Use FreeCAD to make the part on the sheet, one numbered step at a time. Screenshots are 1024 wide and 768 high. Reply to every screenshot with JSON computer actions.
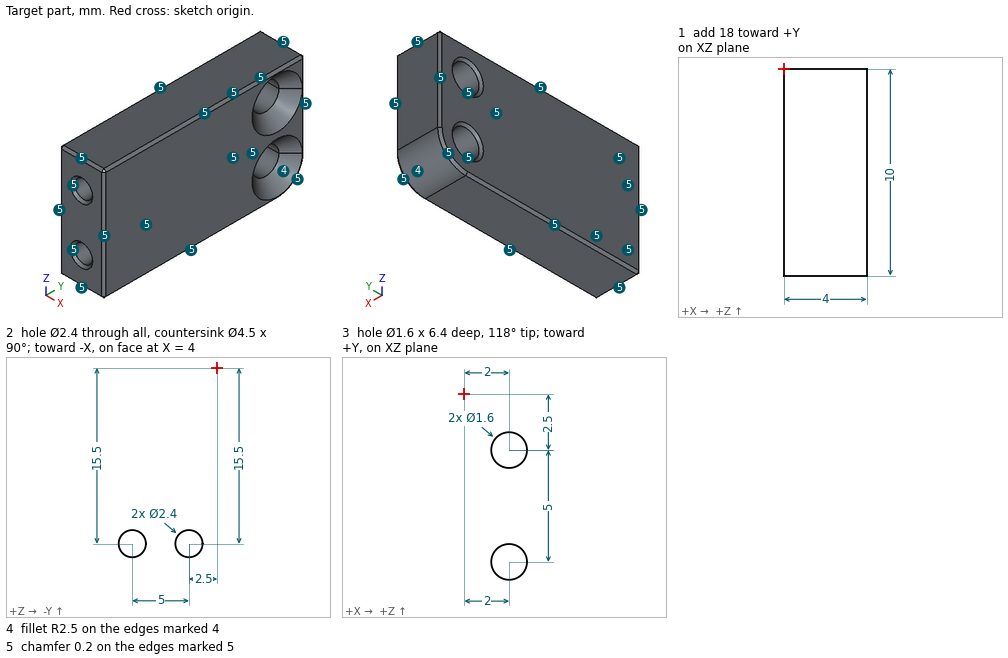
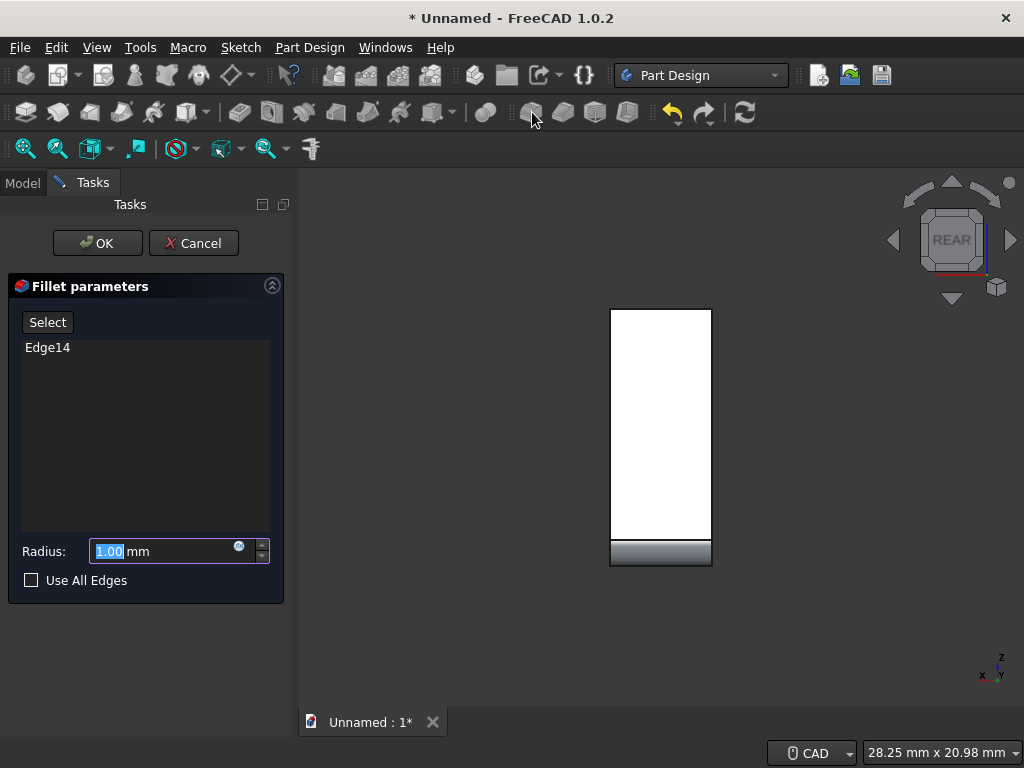
{"action": "type", "text": "2.5"}
{"action": "key", "text": "Tab"}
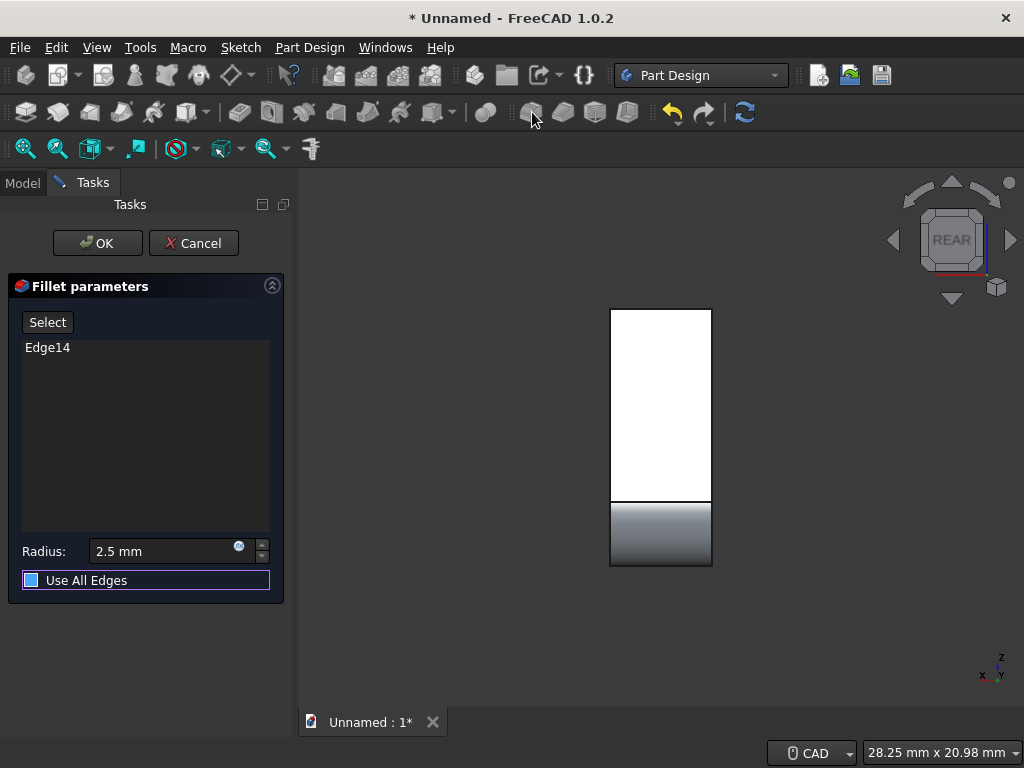
{"action": "left_click", "coordinate": [98, 243]}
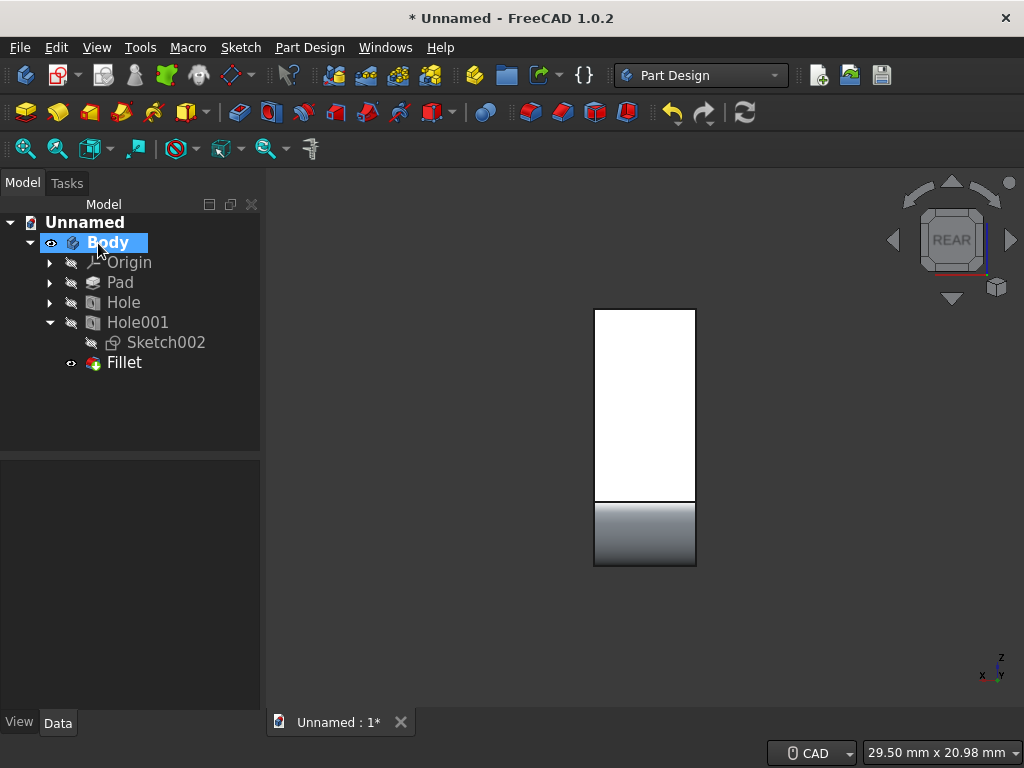
{"action": "left_click", "coordinate": [594, 404]}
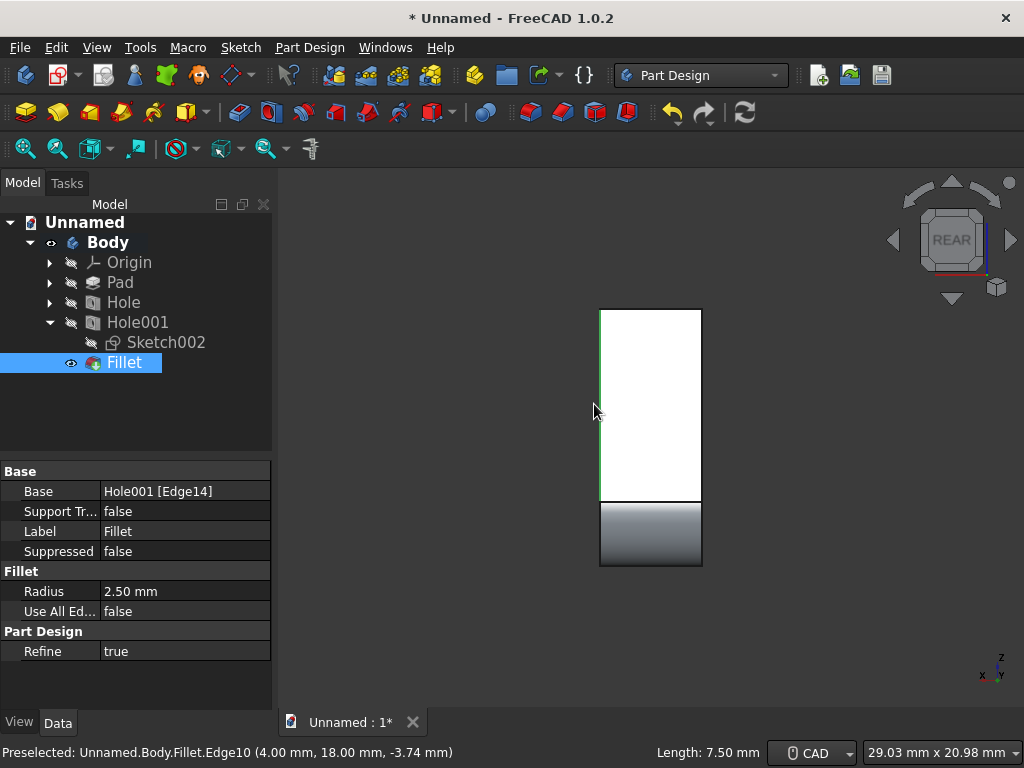
{"action": "left_click", "coordinate": [600, 546], "text": "ctrl"}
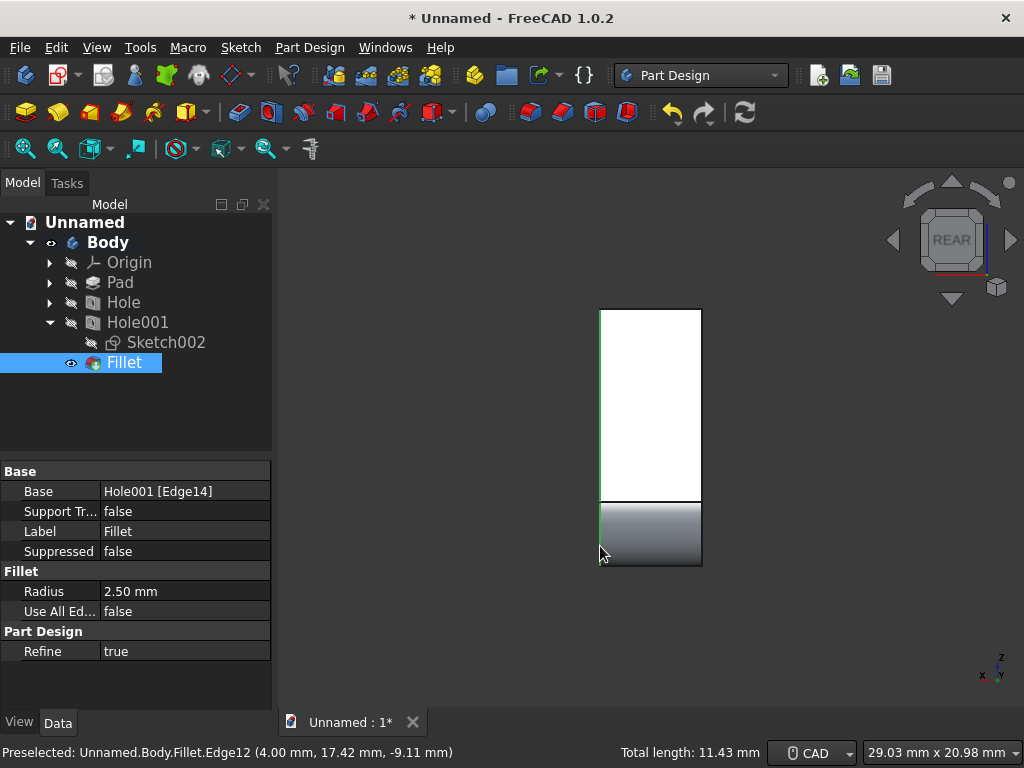
{"action": "key", "text": "0"}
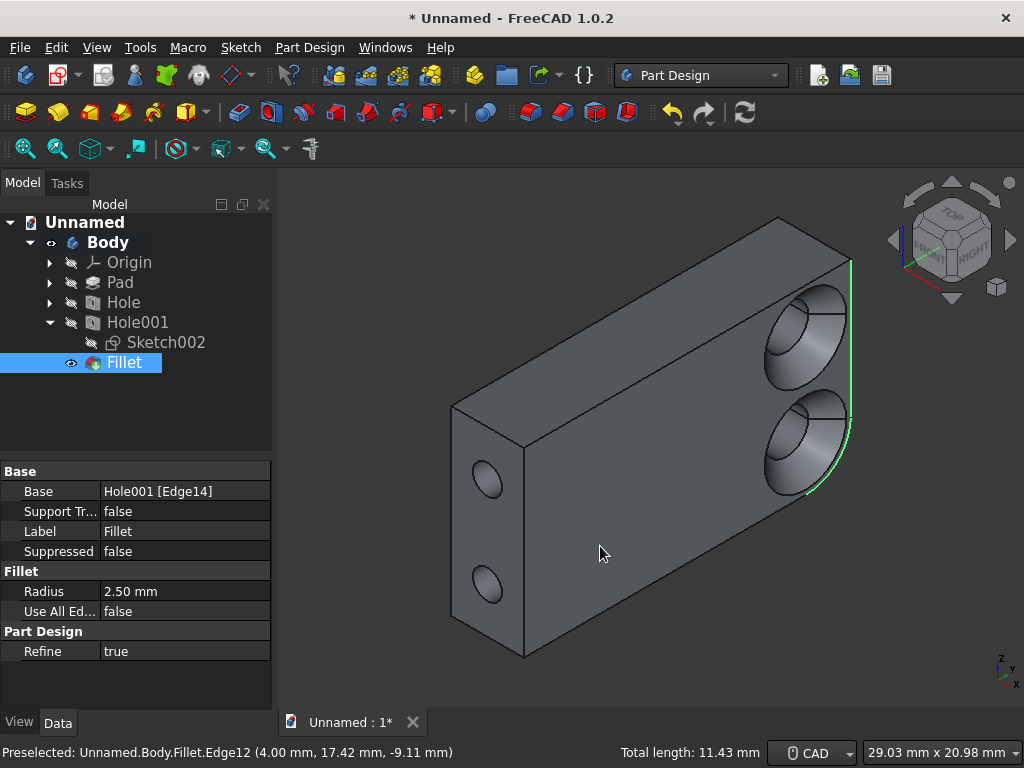
{"action": "left_click", "coordinate": [744, 278], "text": "ctrl"}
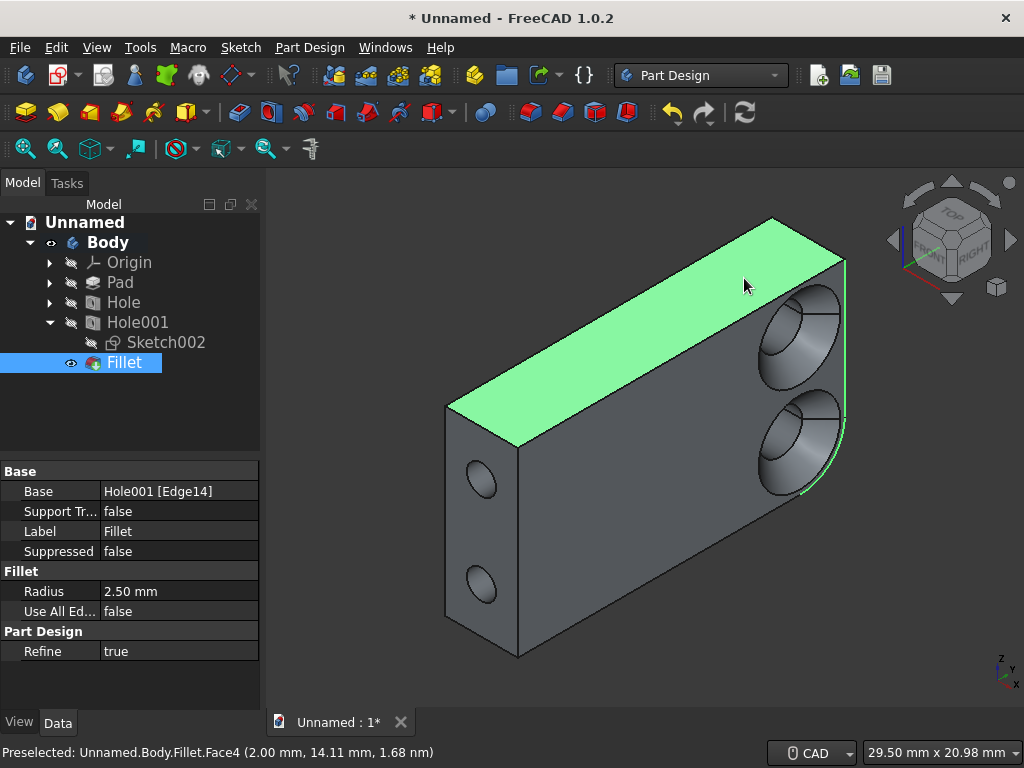
{"action": "left_click", "coordinate": [481, 531], "text": "ctrl"}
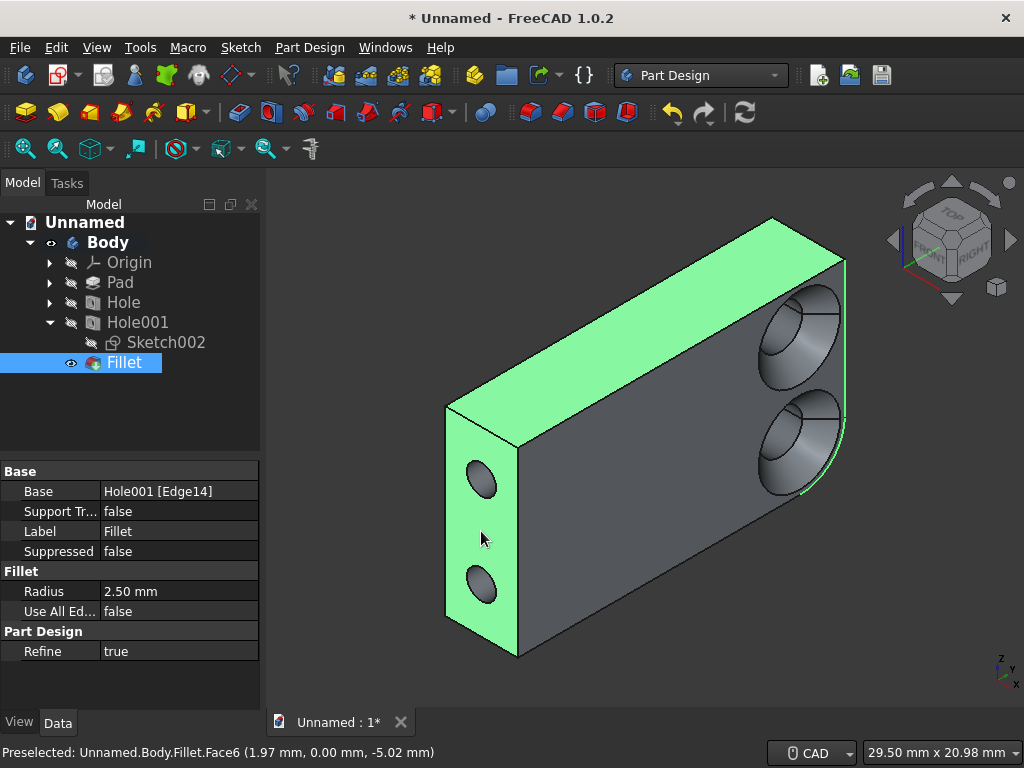
{"action": "key", "text": "2"}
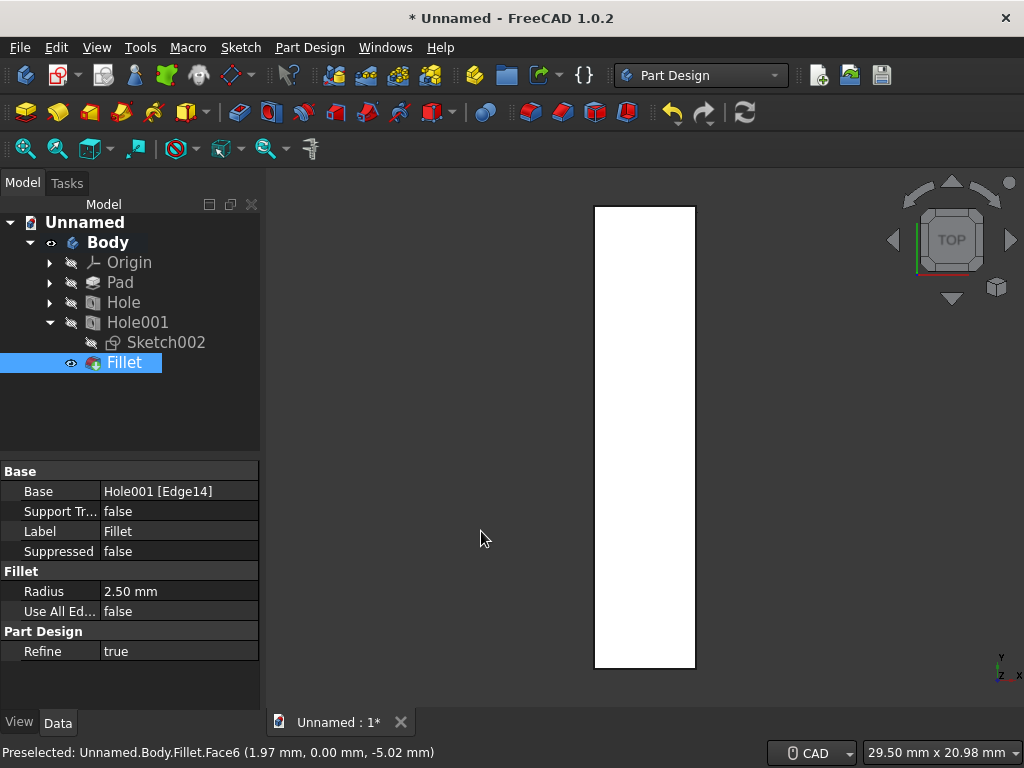
{"action": "key", "text": "1"}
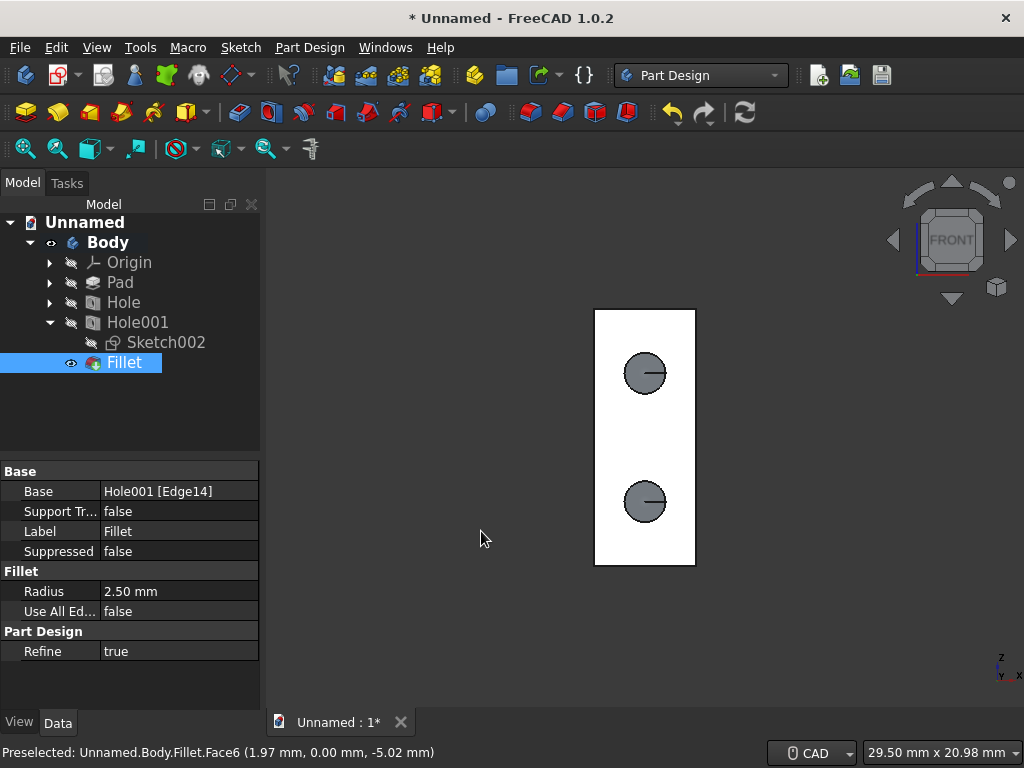
{"action": "key", "text": "3"}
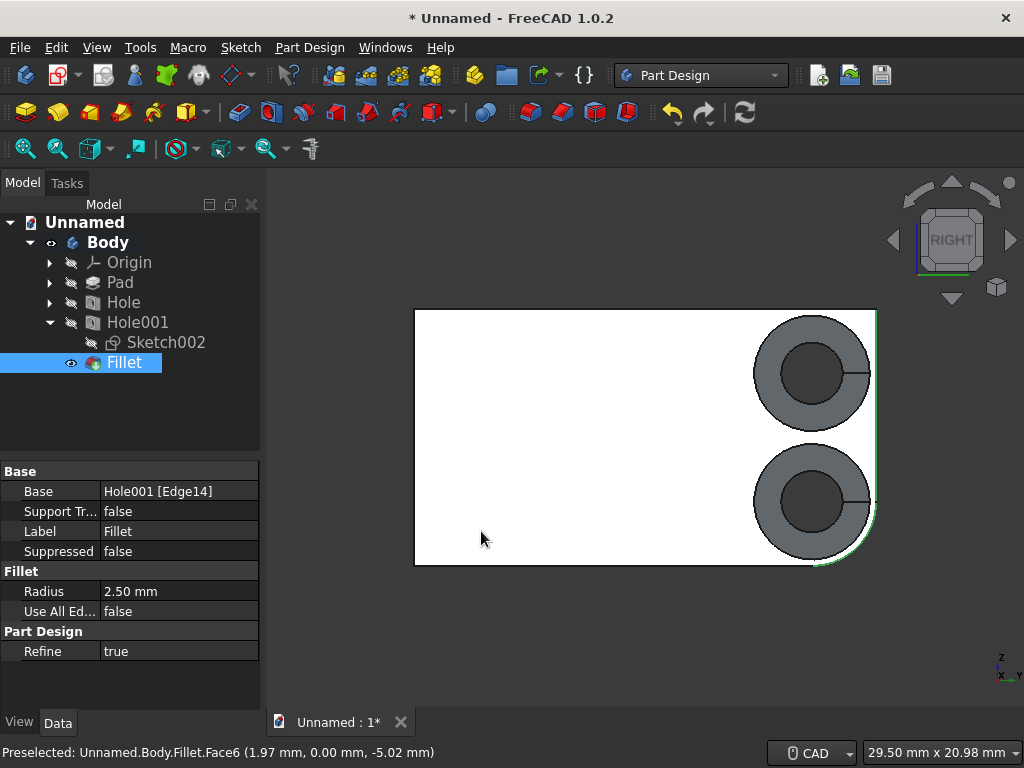
{"action": "left_click", "coordinate": [613, 565], "text": "ctrl"}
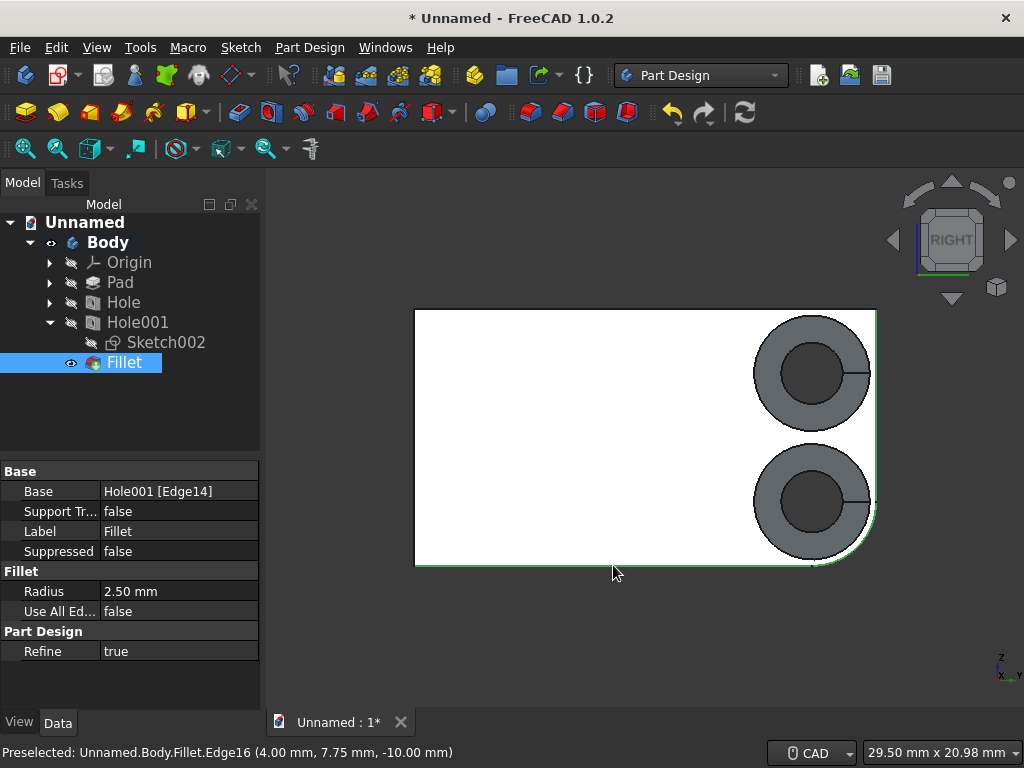
{"action": "key", "text": "5"}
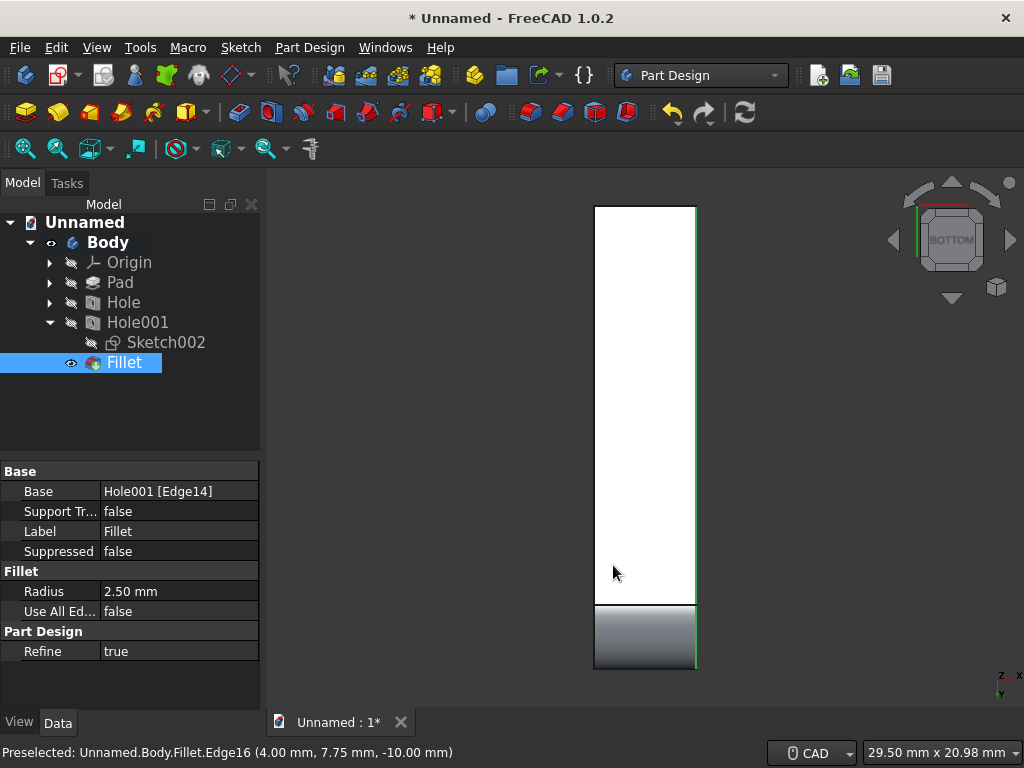
{"action": "key", "text": "4"}